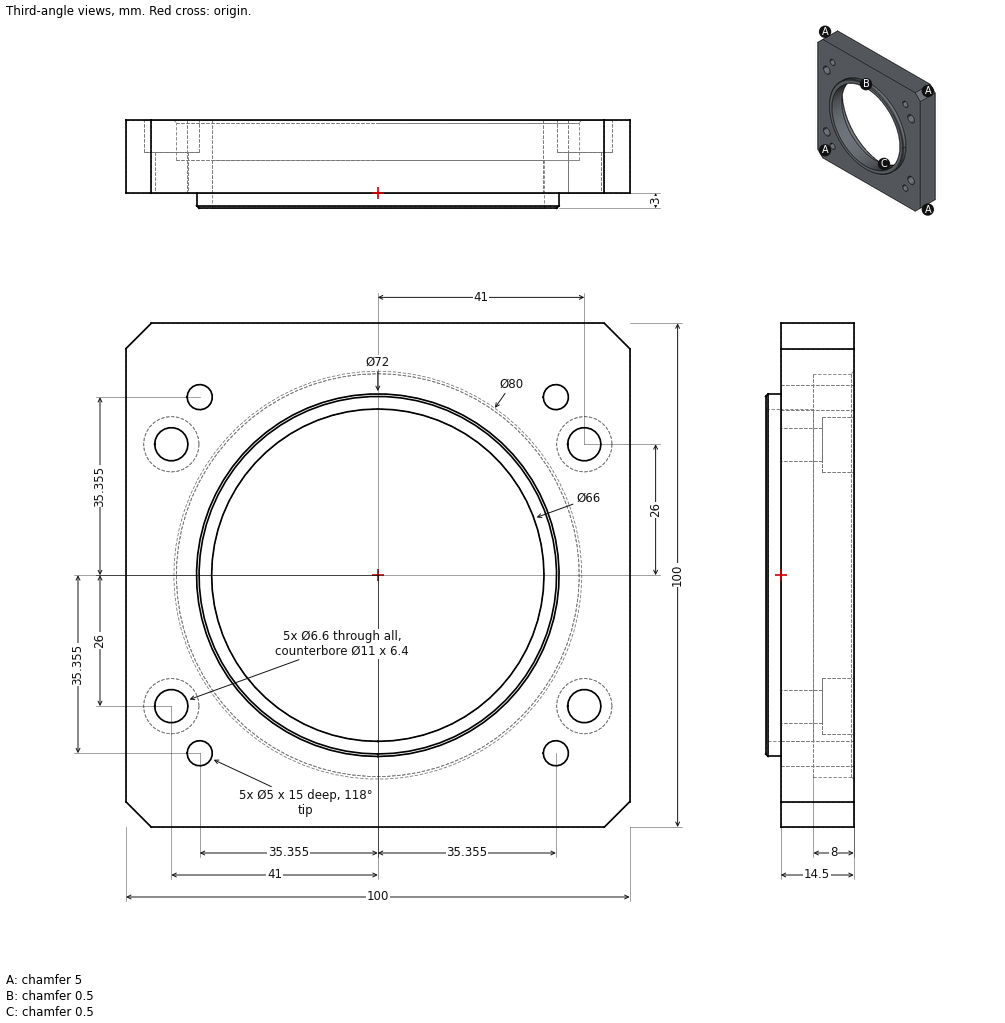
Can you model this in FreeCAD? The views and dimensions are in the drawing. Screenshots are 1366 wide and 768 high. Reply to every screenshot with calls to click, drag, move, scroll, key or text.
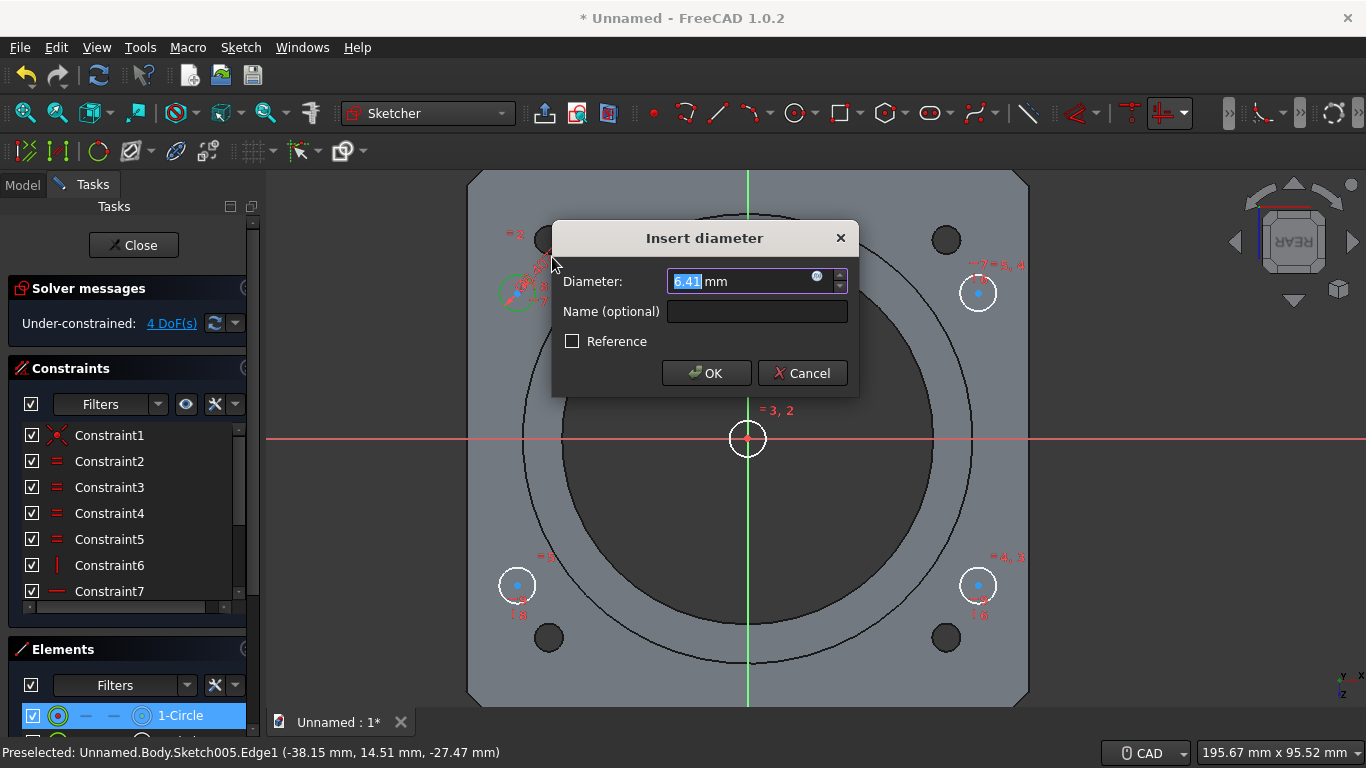
text(6.6)
key(Return)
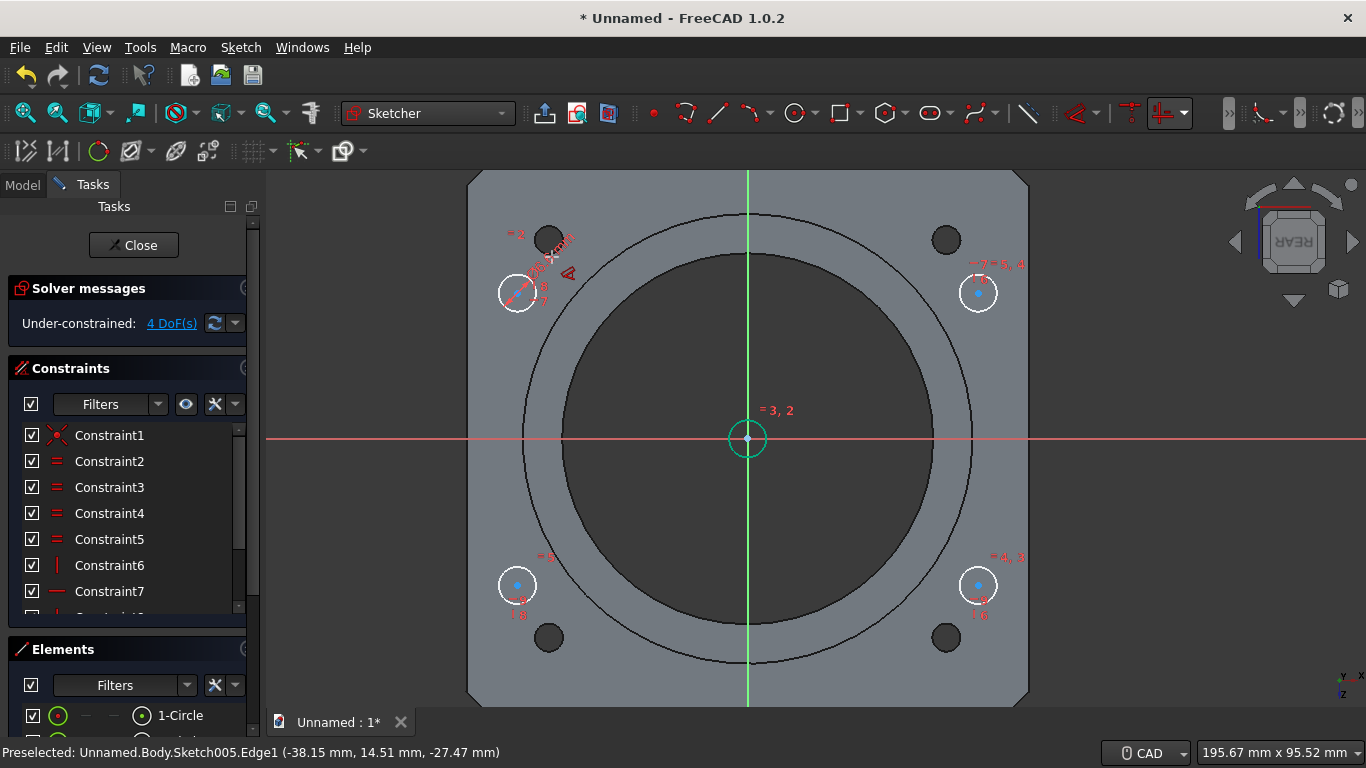
click(517, 293)
click(633, 259)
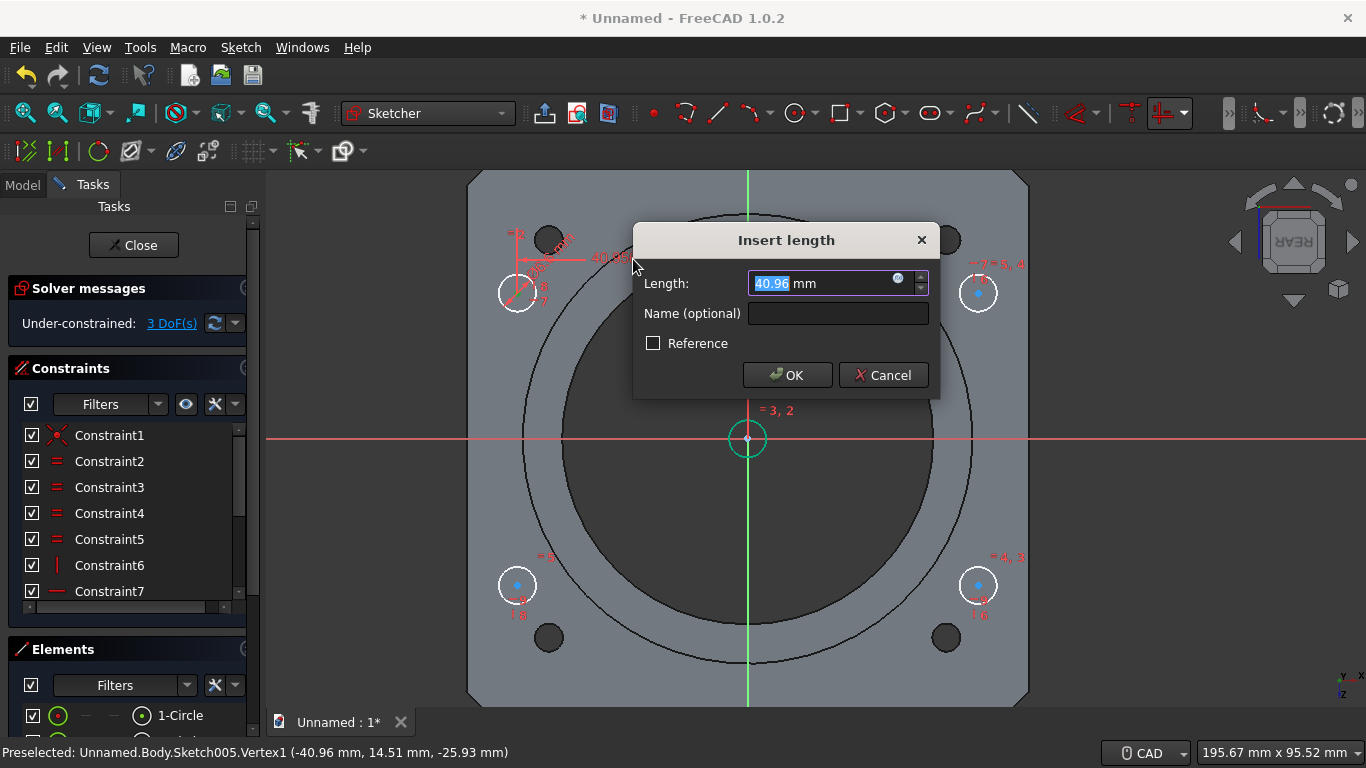
text(41)
key(Return)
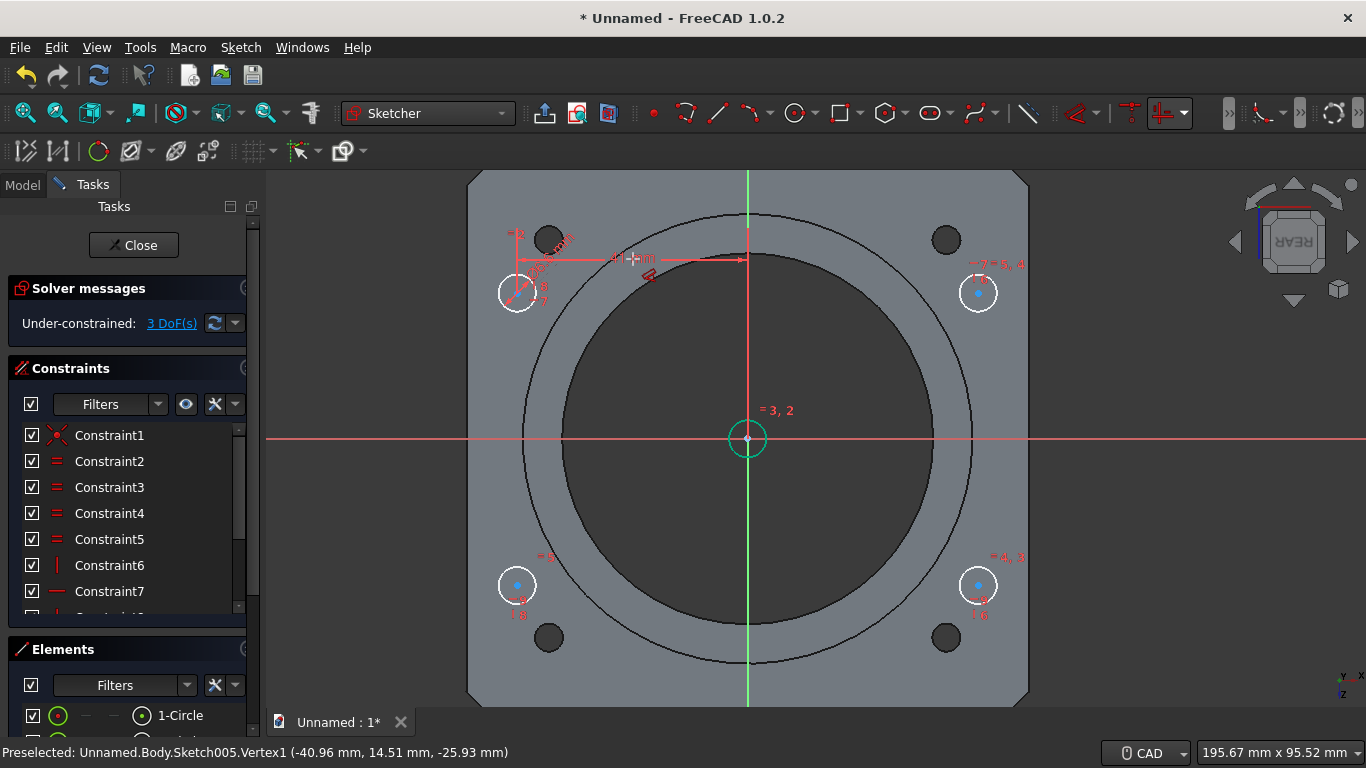
click(517, 293)
click(483, 366)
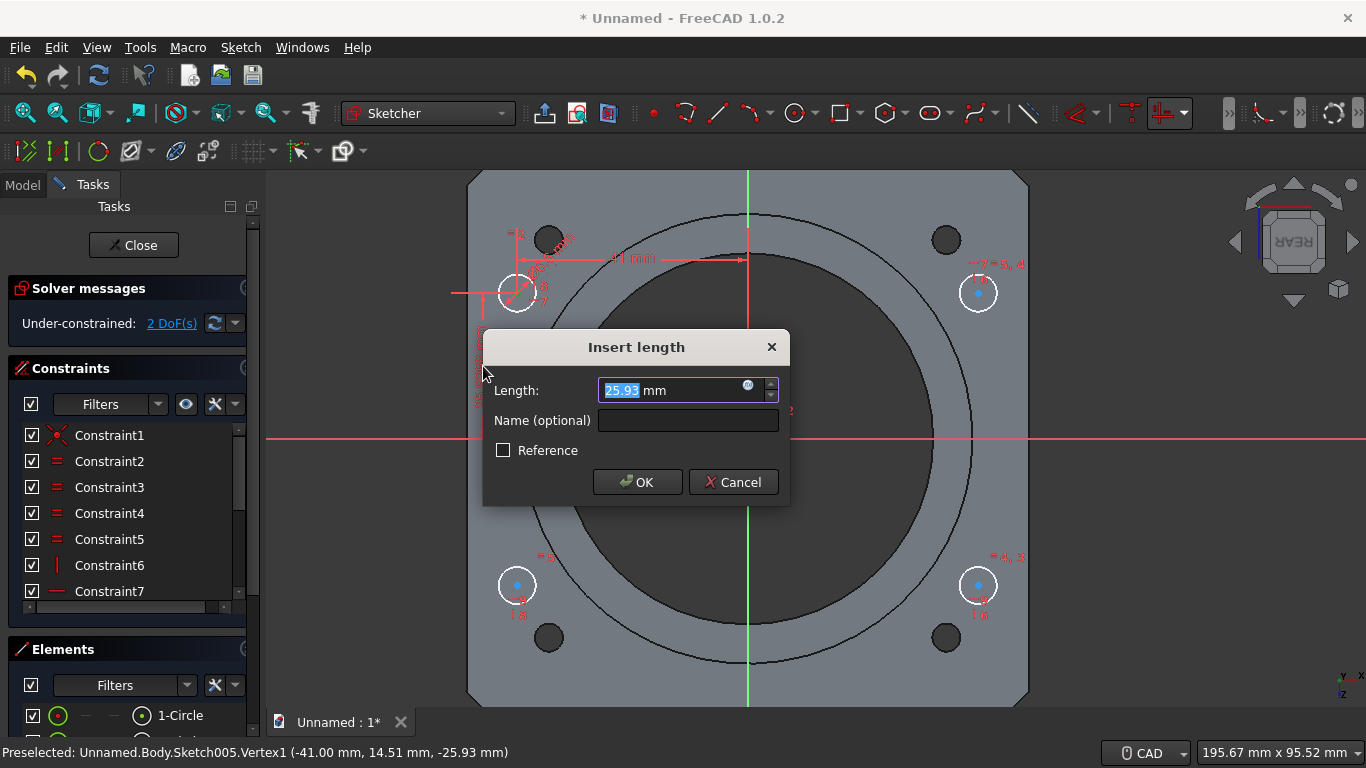
text(26)
key(Return)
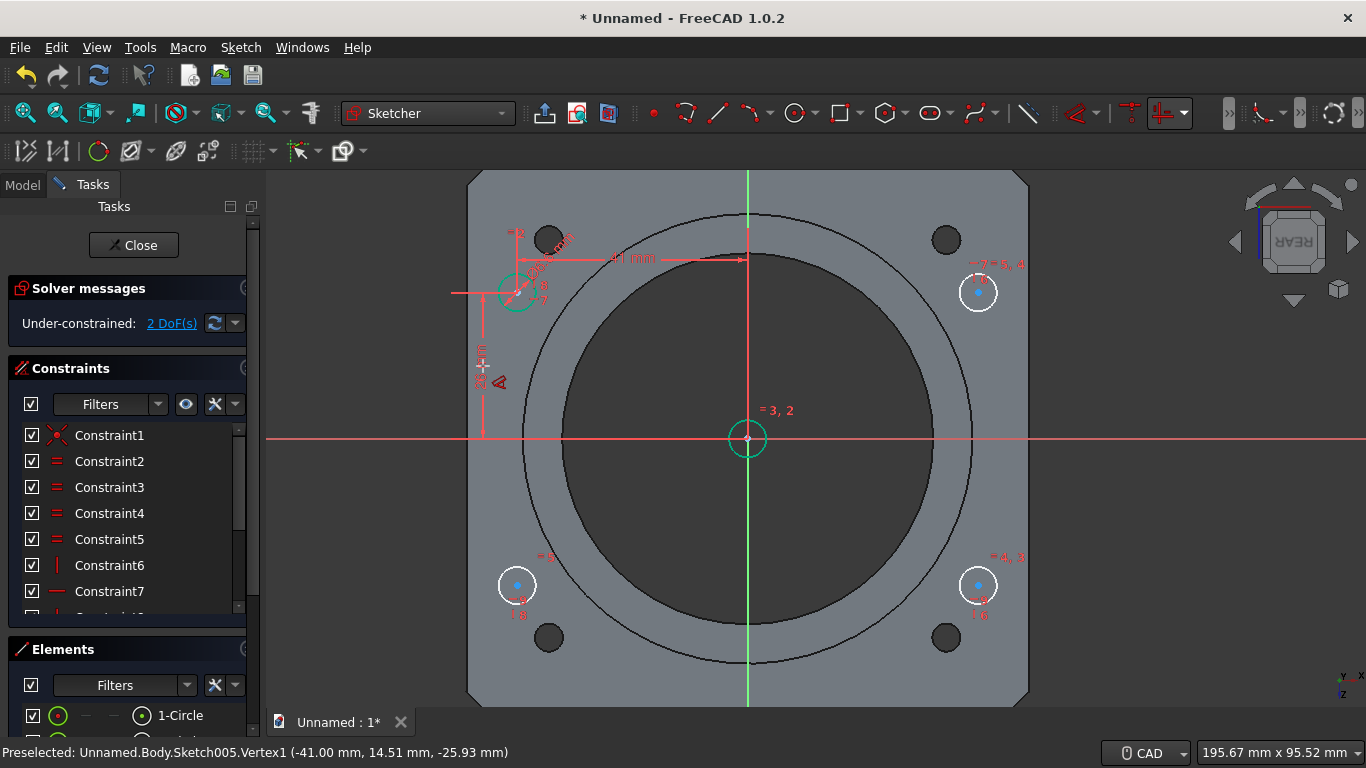
click(978, 586)
click(863, 620)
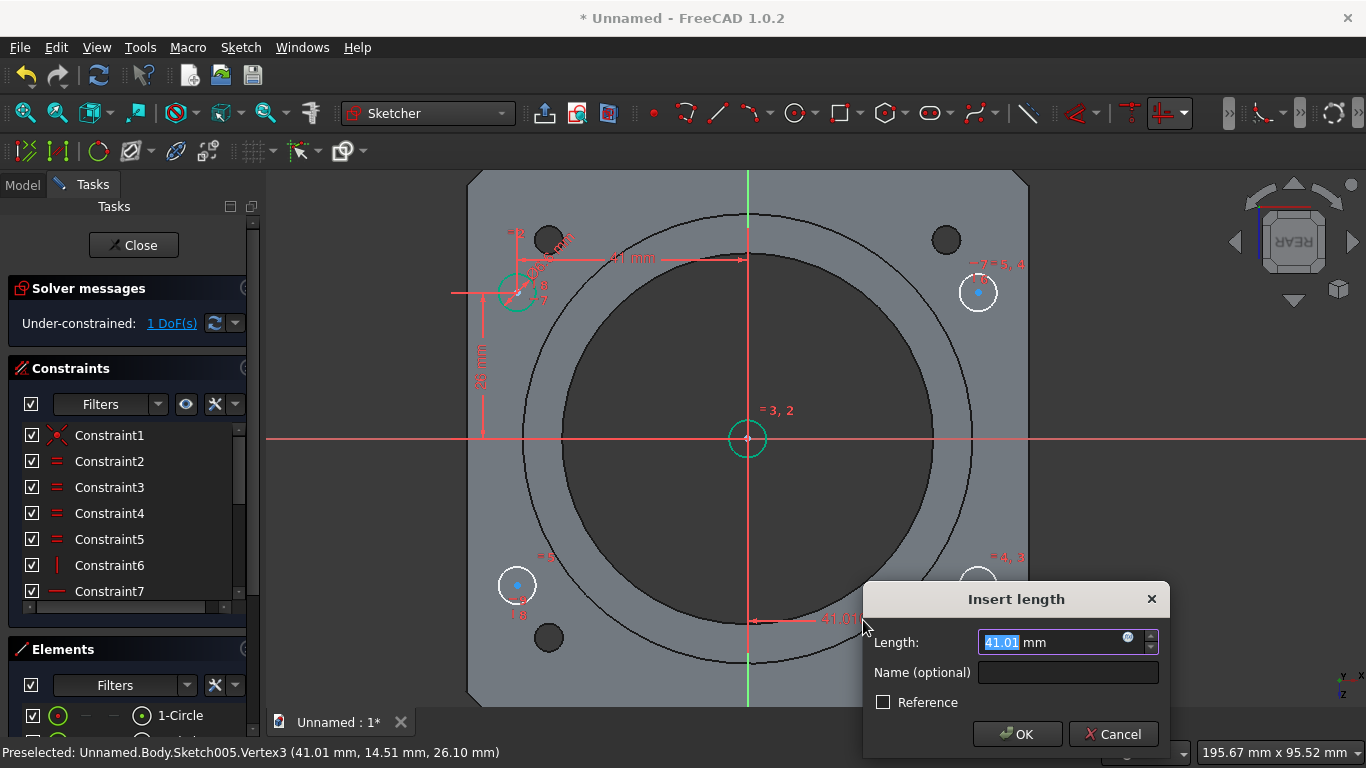
text(41)
key(Return)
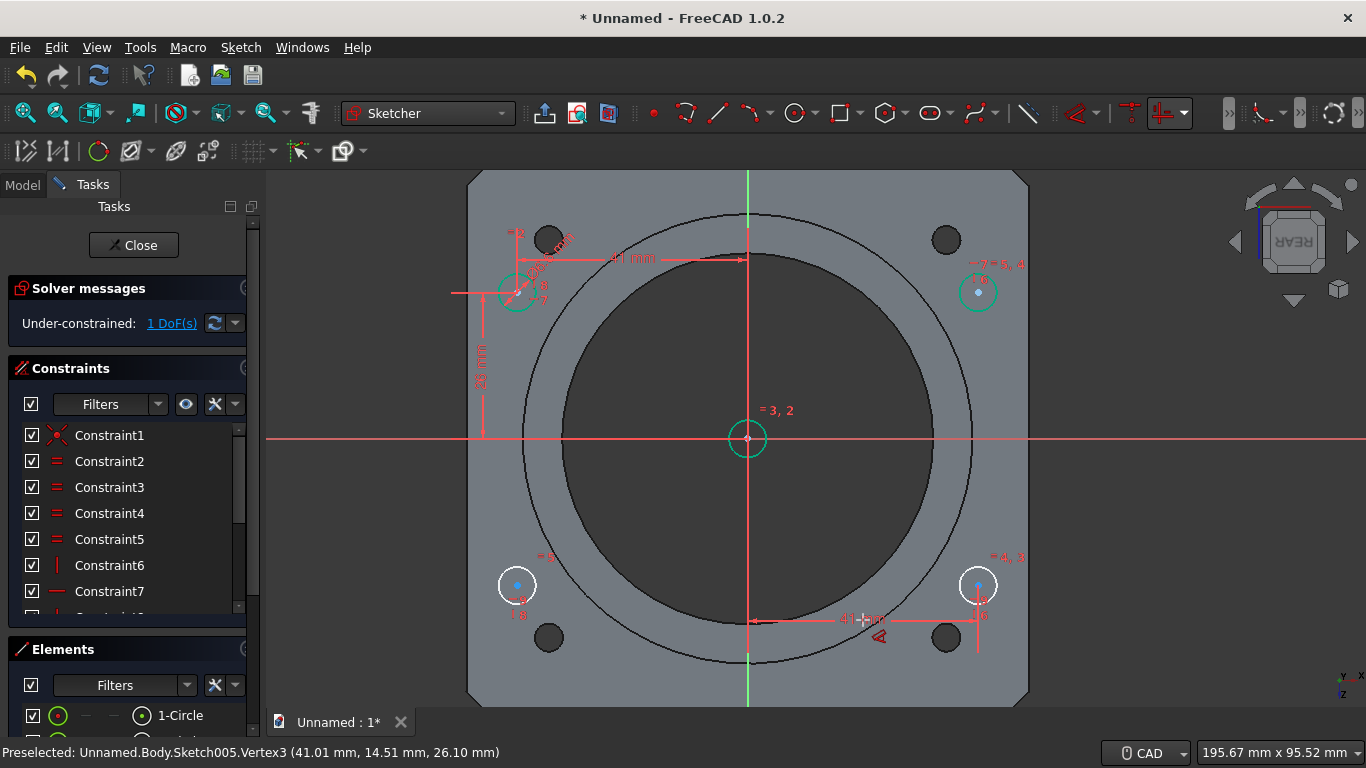
click(978, 586)
click(1012, 512)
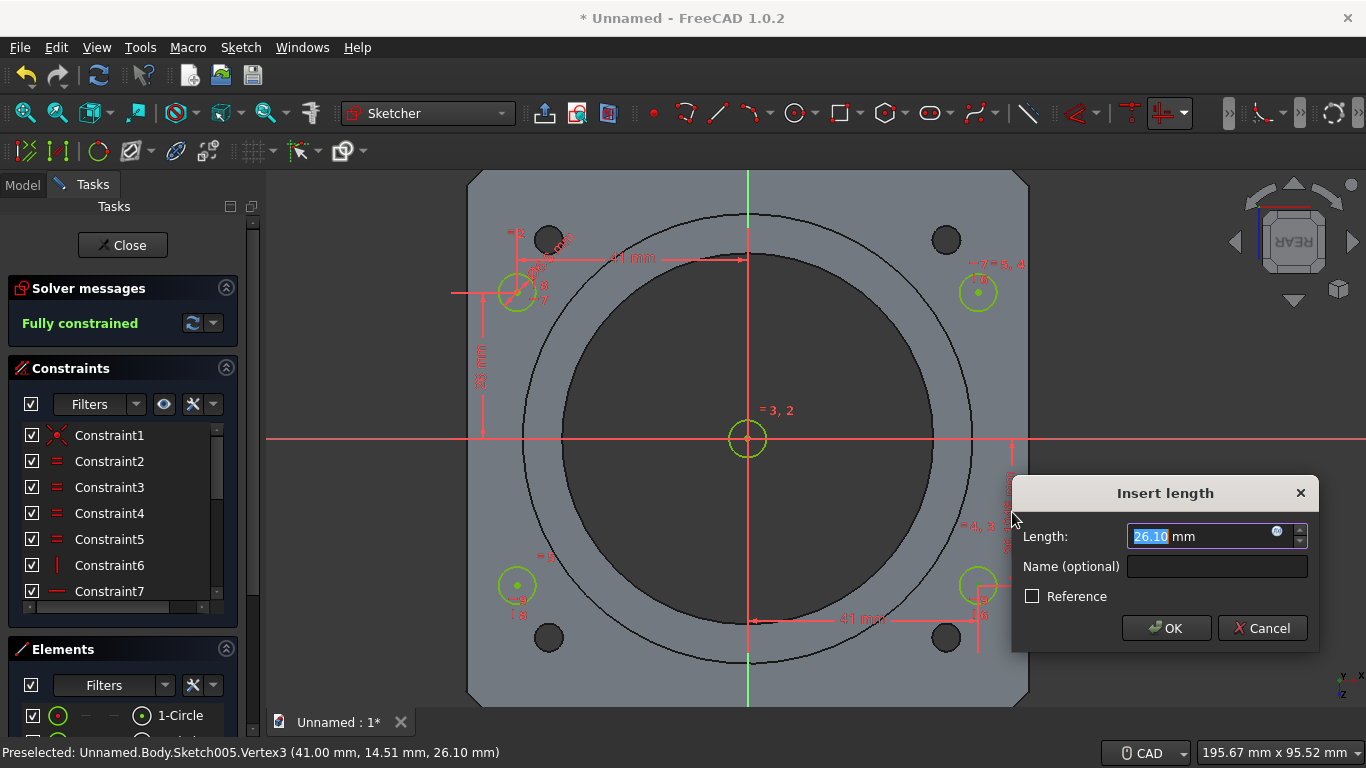
text(26)
key(Return)
key(Escape)